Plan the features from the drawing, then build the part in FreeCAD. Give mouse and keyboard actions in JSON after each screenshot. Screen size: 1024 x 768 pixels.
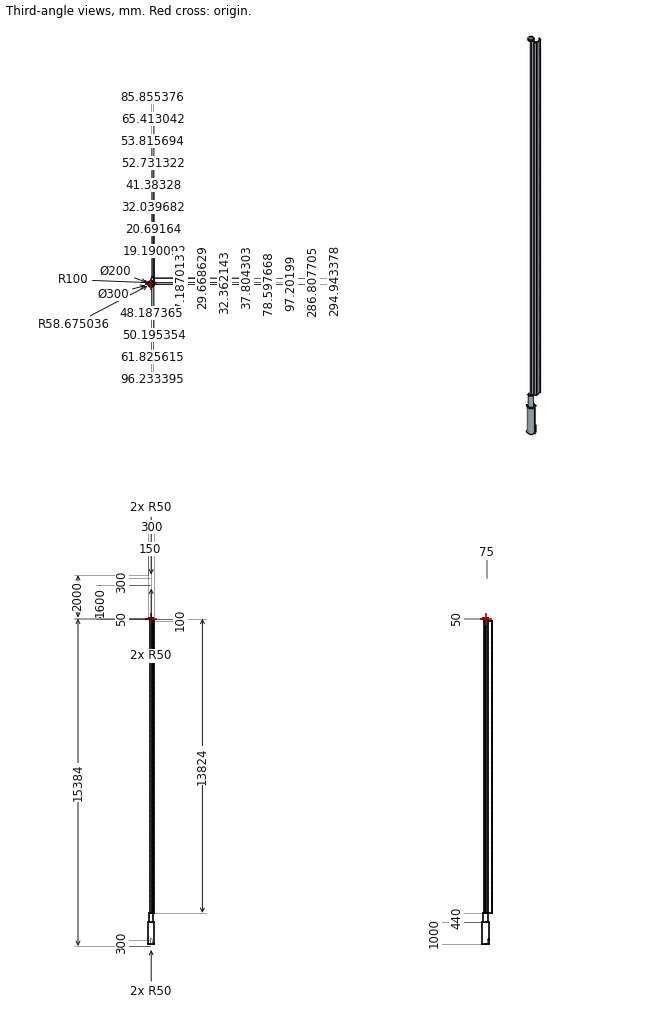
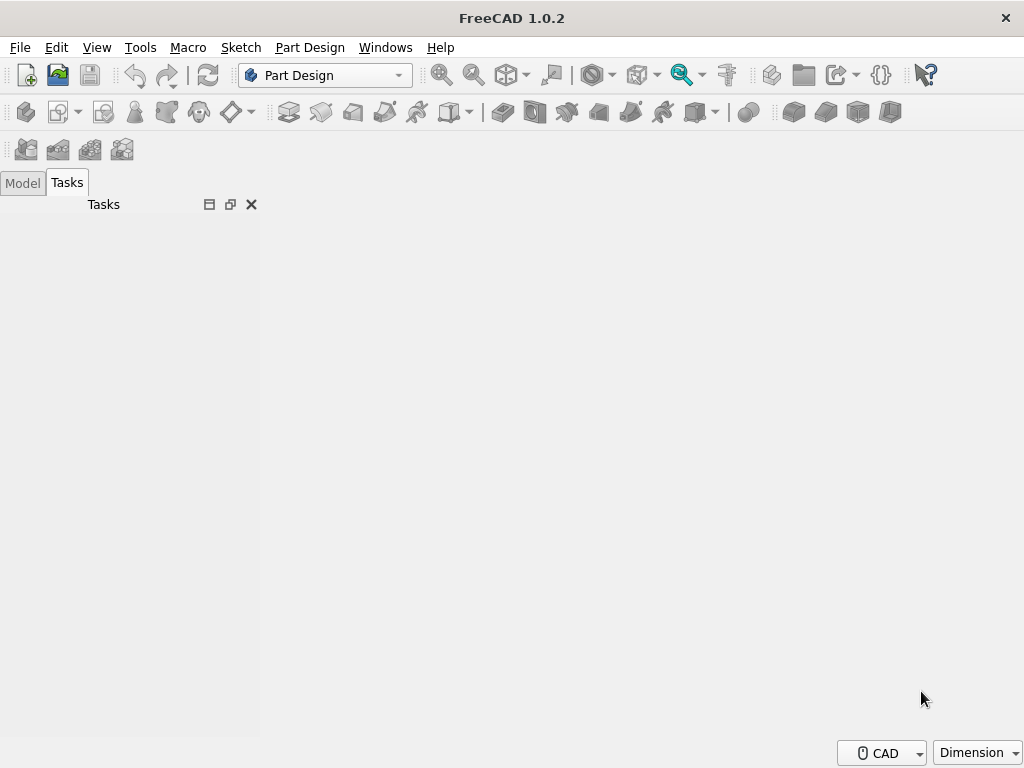
{"action": "left_click", "coordinate": [26, 76]}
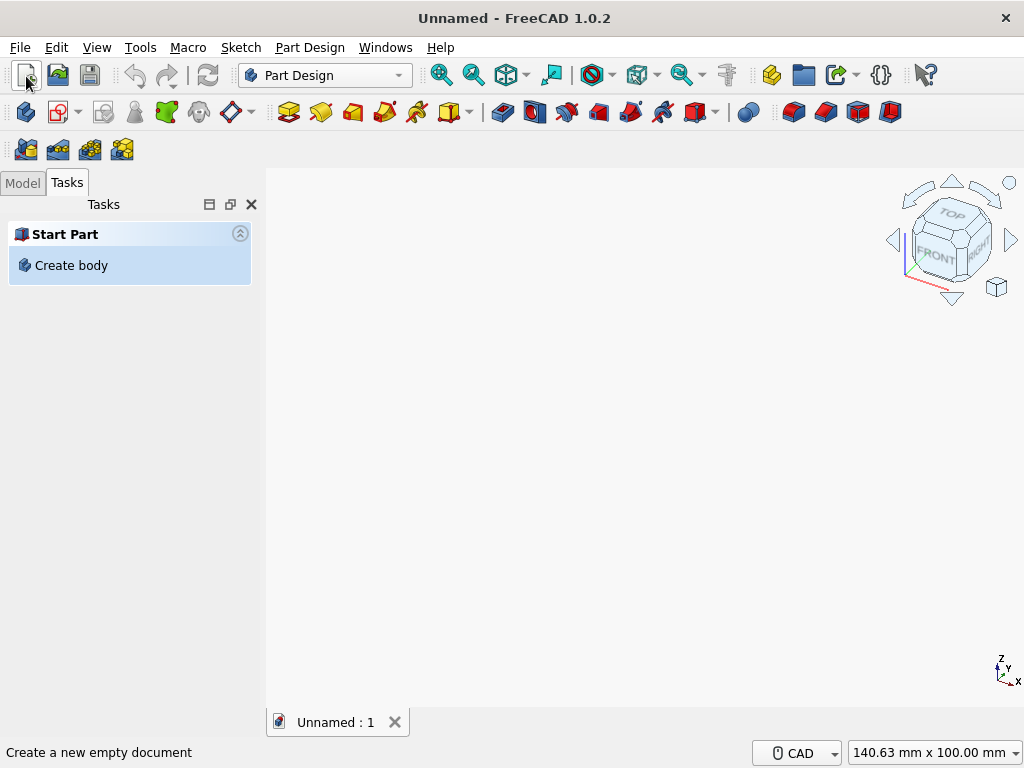
{"action": "left_click", "coordinate": [58, 112]}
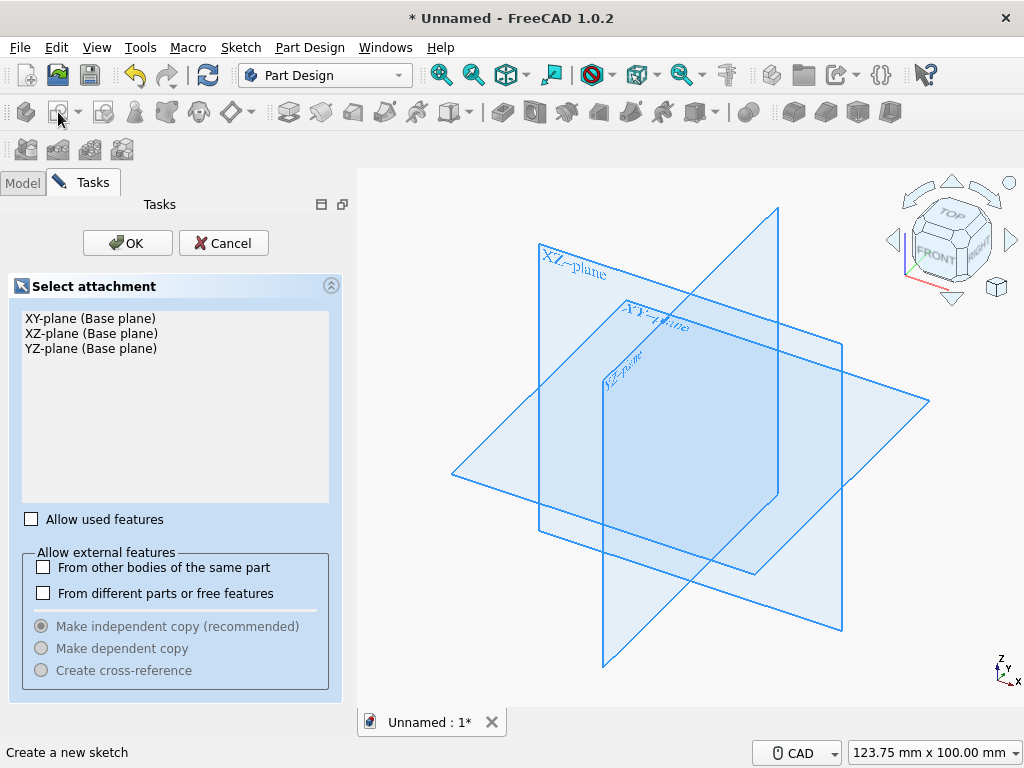
{"action": "left_click", "coordinate": [82, 318]}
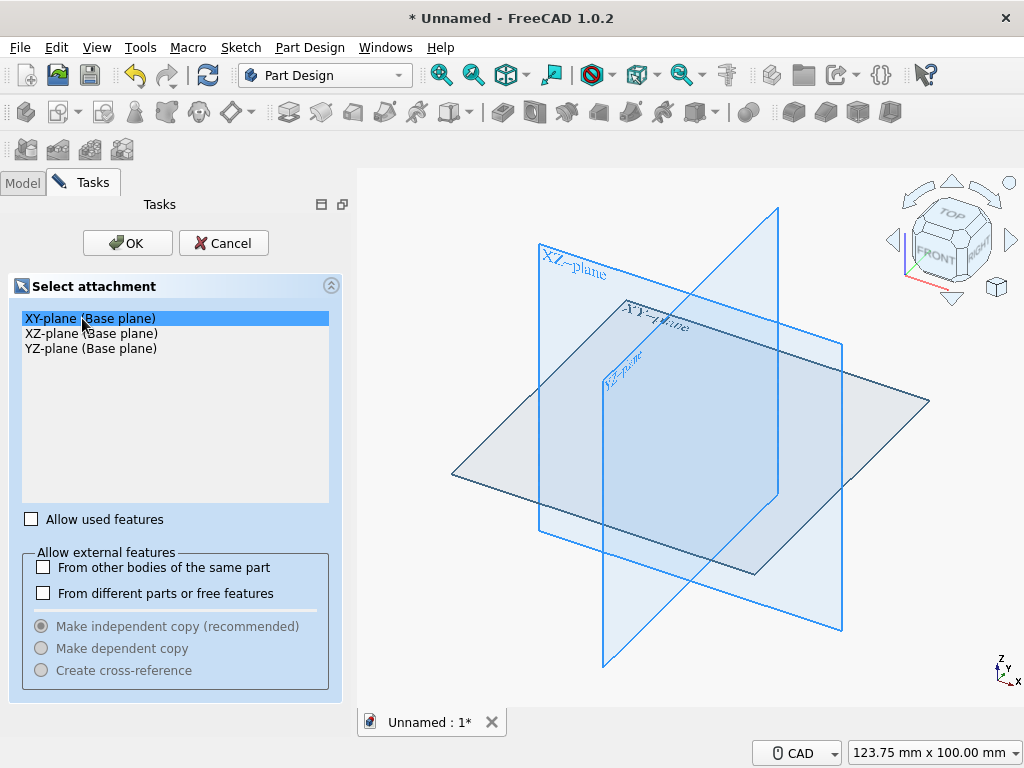
{"action": "left_click", "coordinate": [128, 243]}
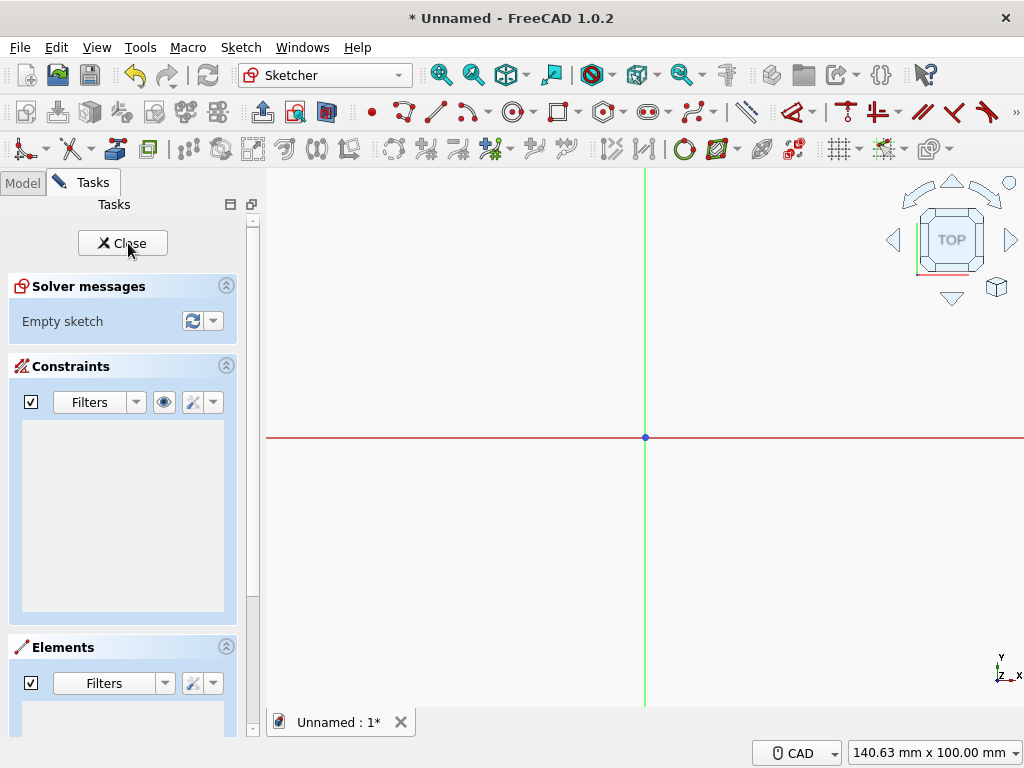
{"action": "scroll", "coordinate": [547, 438], "scroll_direction": "down", "scroll_amount": 6}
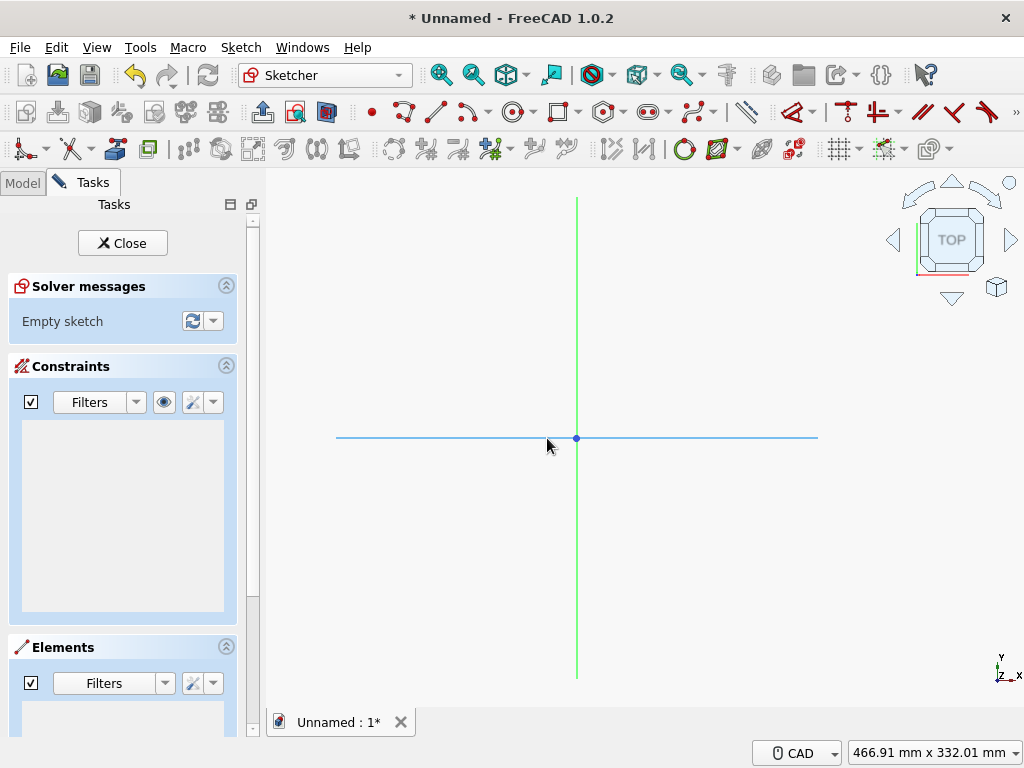
{"action": "left_click", "coordinate": [514, 112]}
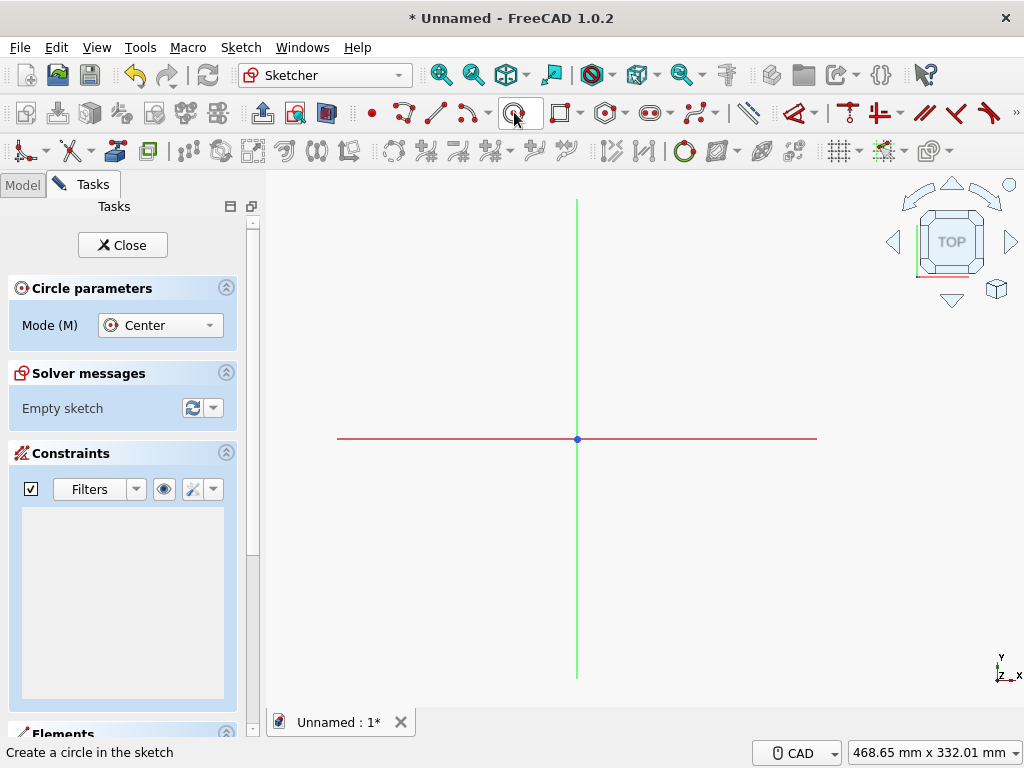
{"action": "left_click", "coordinate": [577, 439]}
{"action": "left_click", "coordinate": [691, 325]}
{"action": "key", "text": "Escape"}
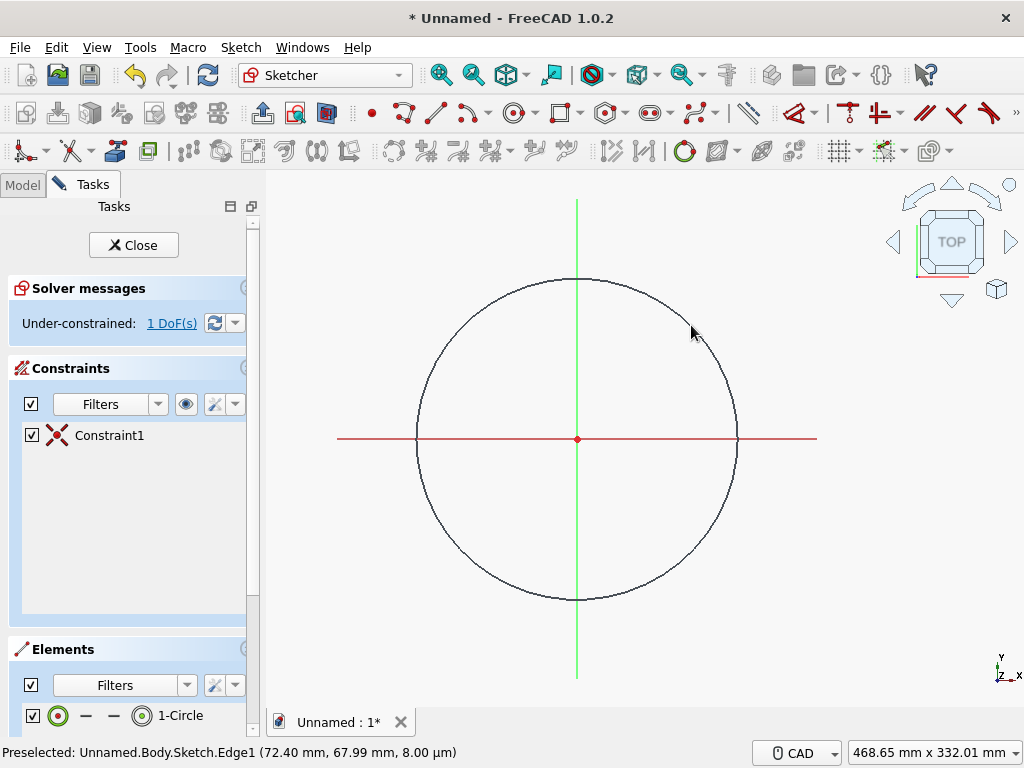
{"action": "left_click", "coordinate": [794, 114]}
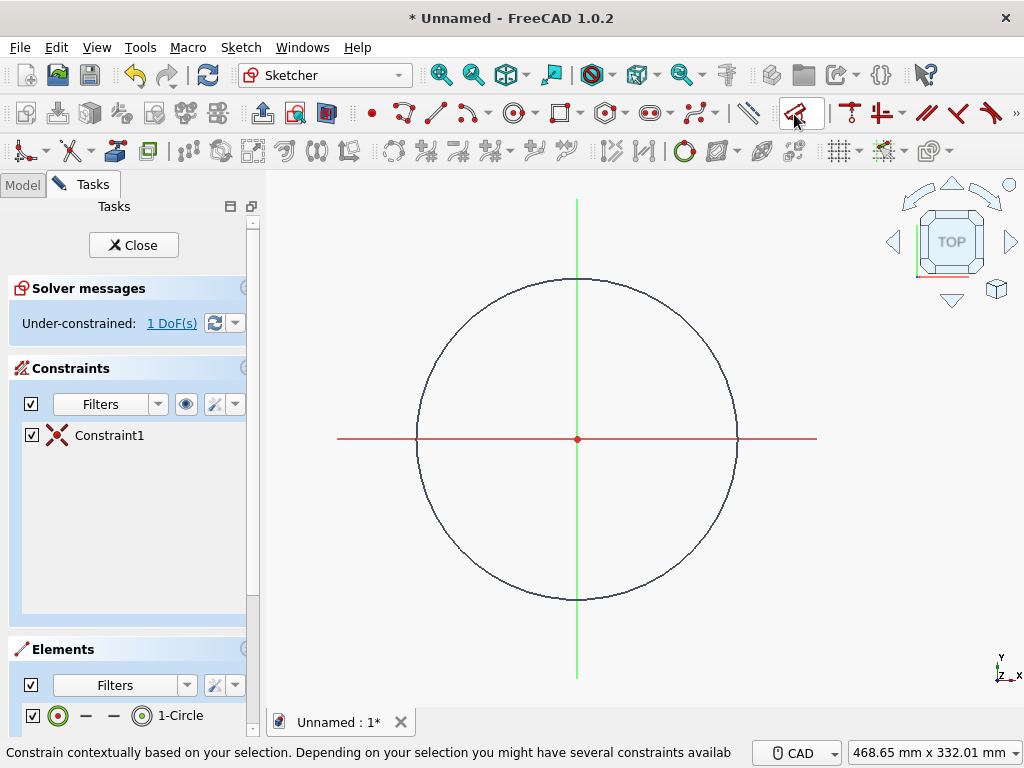
{"action": "left_click", "coordinate": [690, 325]}
{"action": "left_click", "coordinate": [713, 302]}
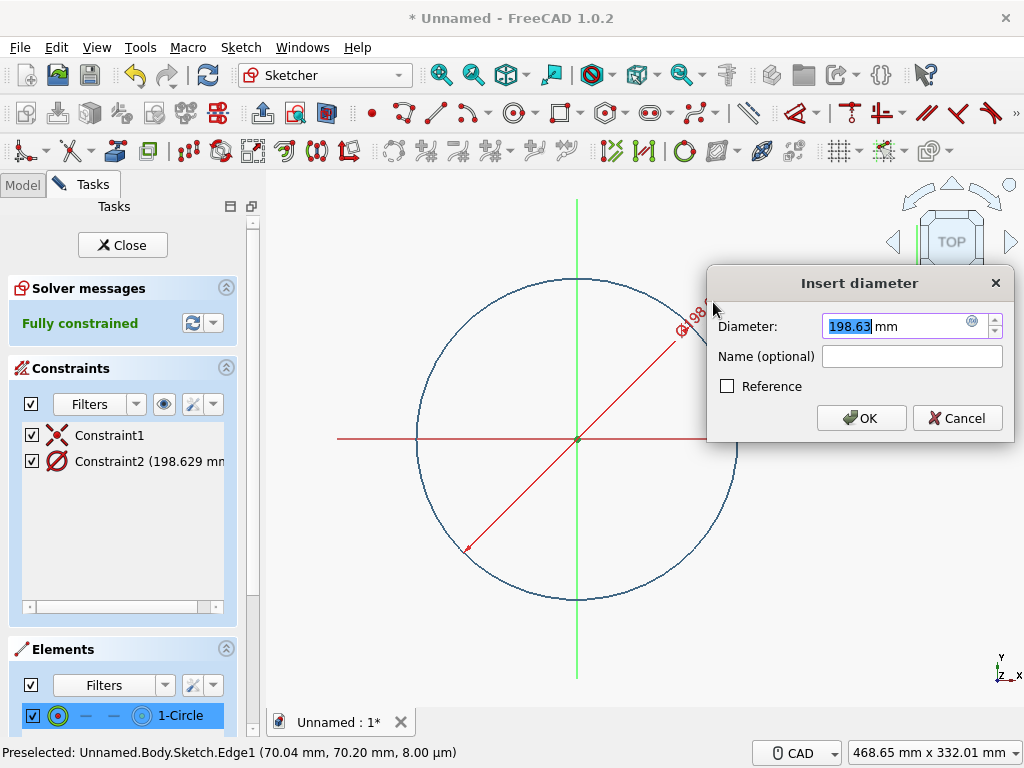
{"action": "type", "text": "200"}
{"action": "key", "text": "Return"}
{"action": "key", "text": "Escape"}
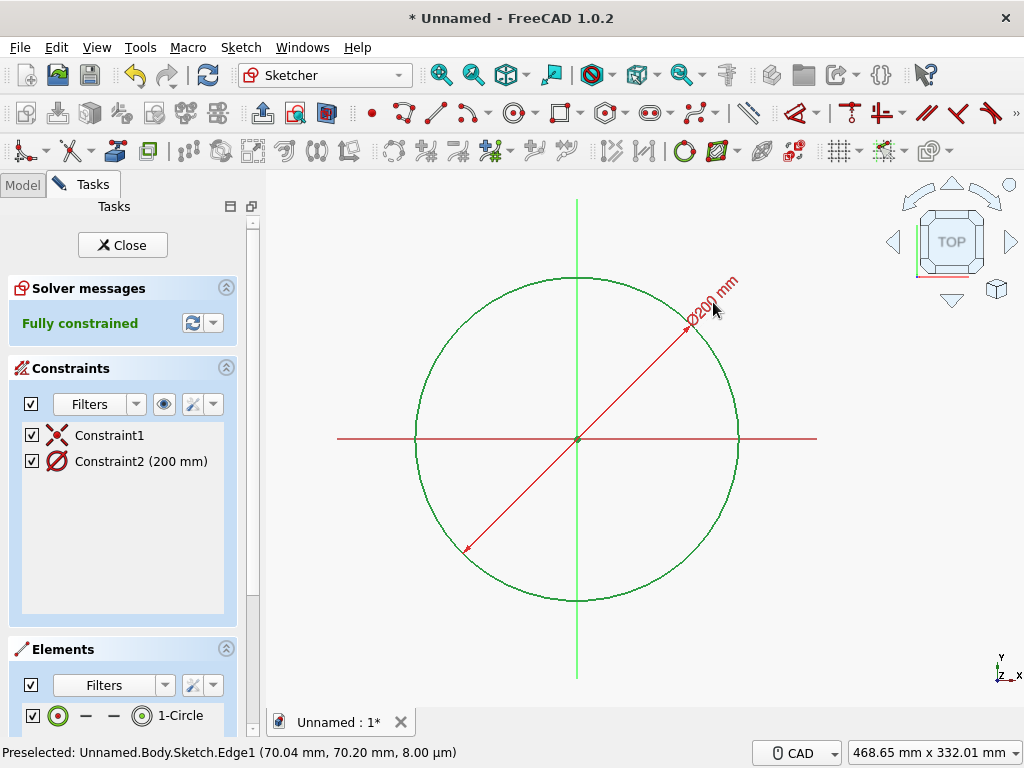
{"action": "left_click", "coordinate": [123, 245]}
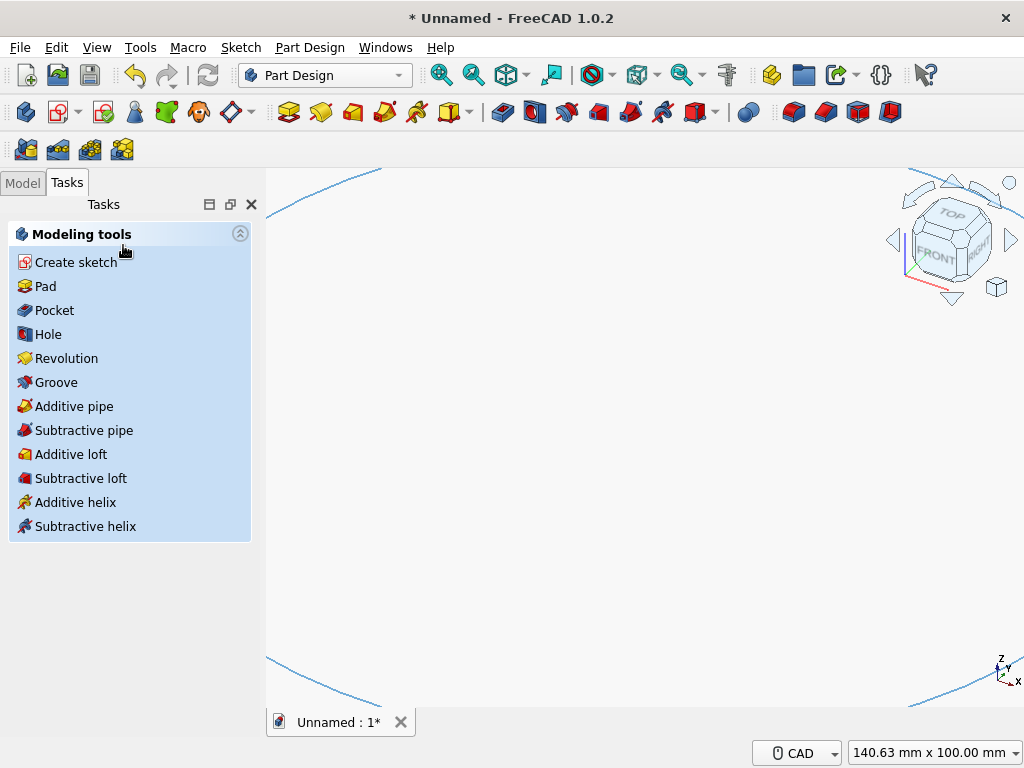
{"action": "left_click", "coordinate": [290, 112]}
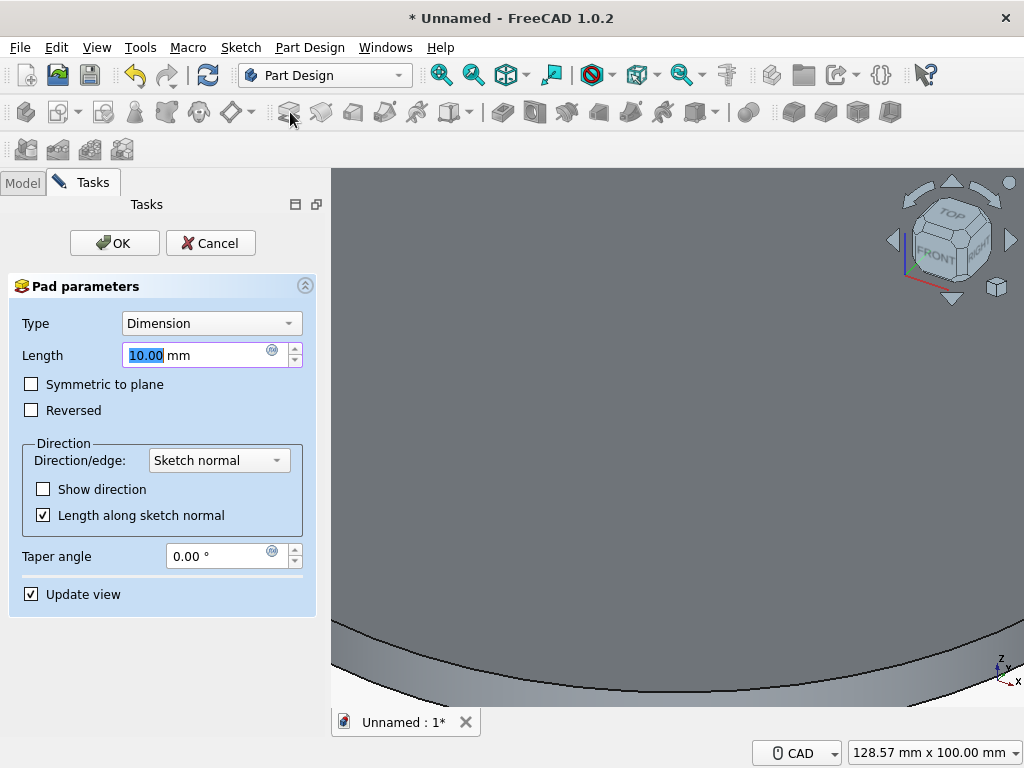
{"action": "type", "text": "50"}
{"action": "key", "text": "Tab"}